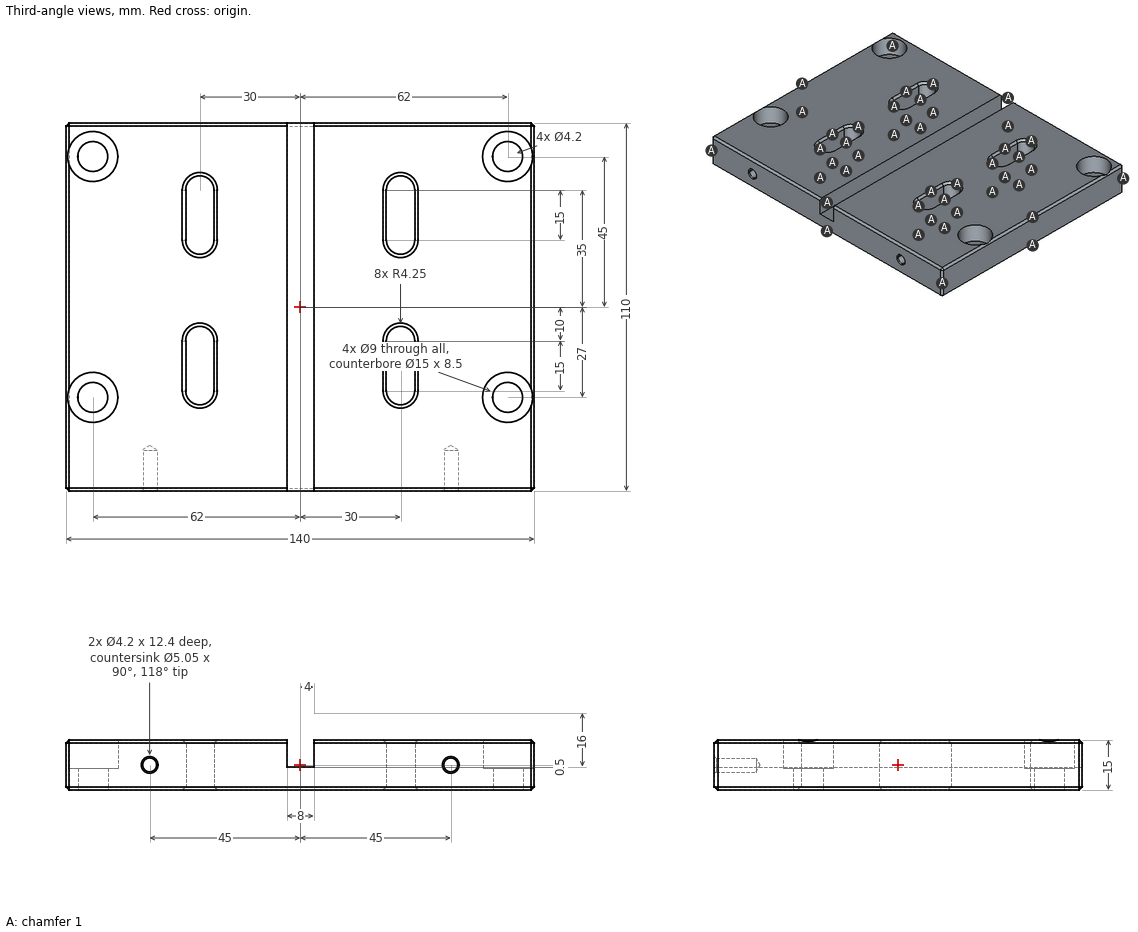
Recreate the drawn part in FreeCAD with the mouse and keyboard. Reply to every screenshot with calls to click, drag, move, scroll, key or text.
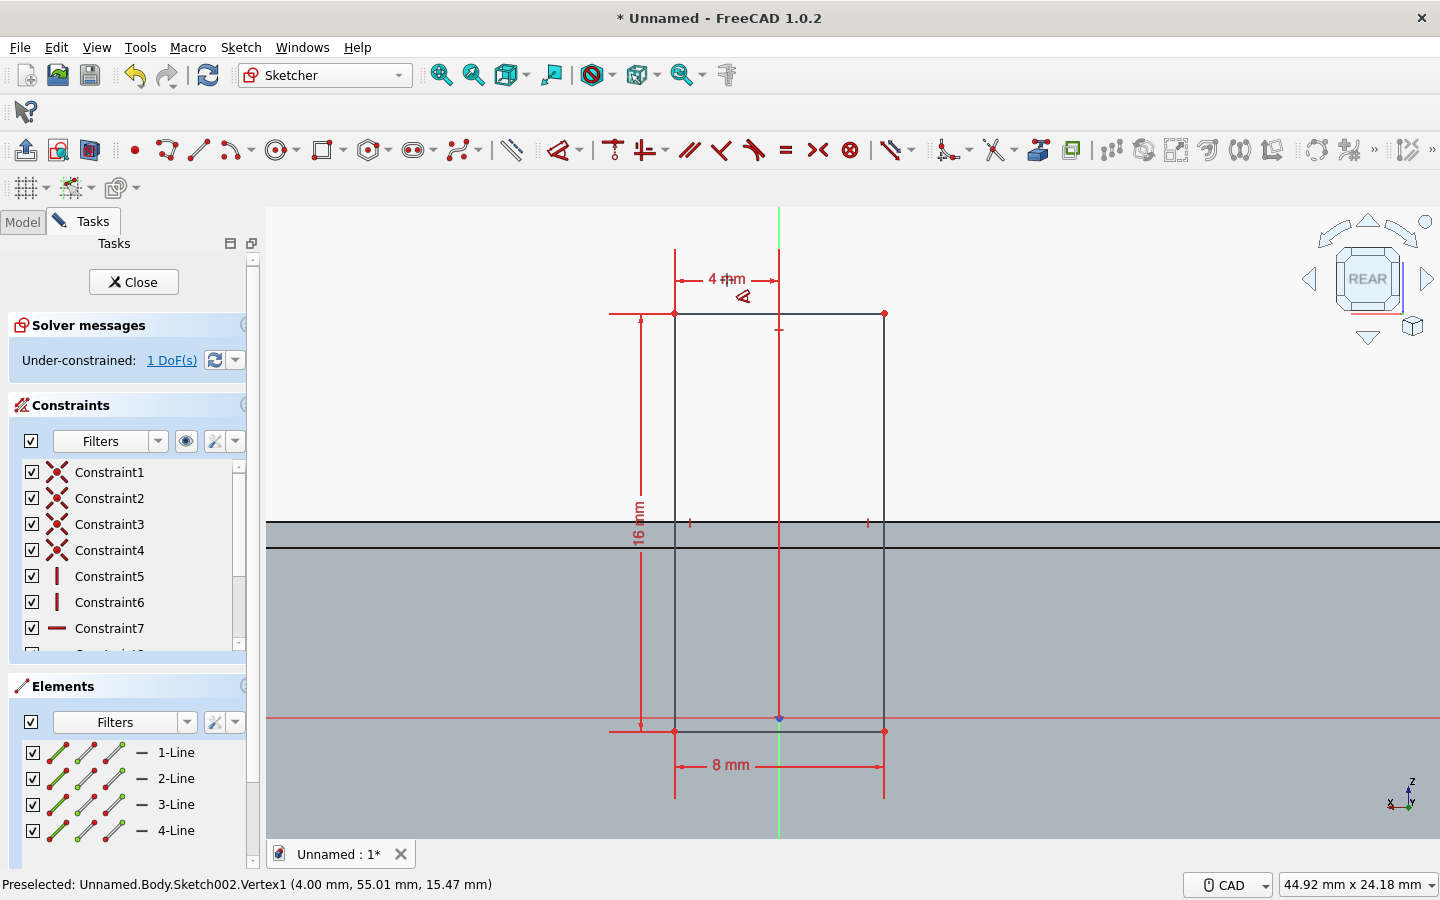
scroll(675, 732, up, 6)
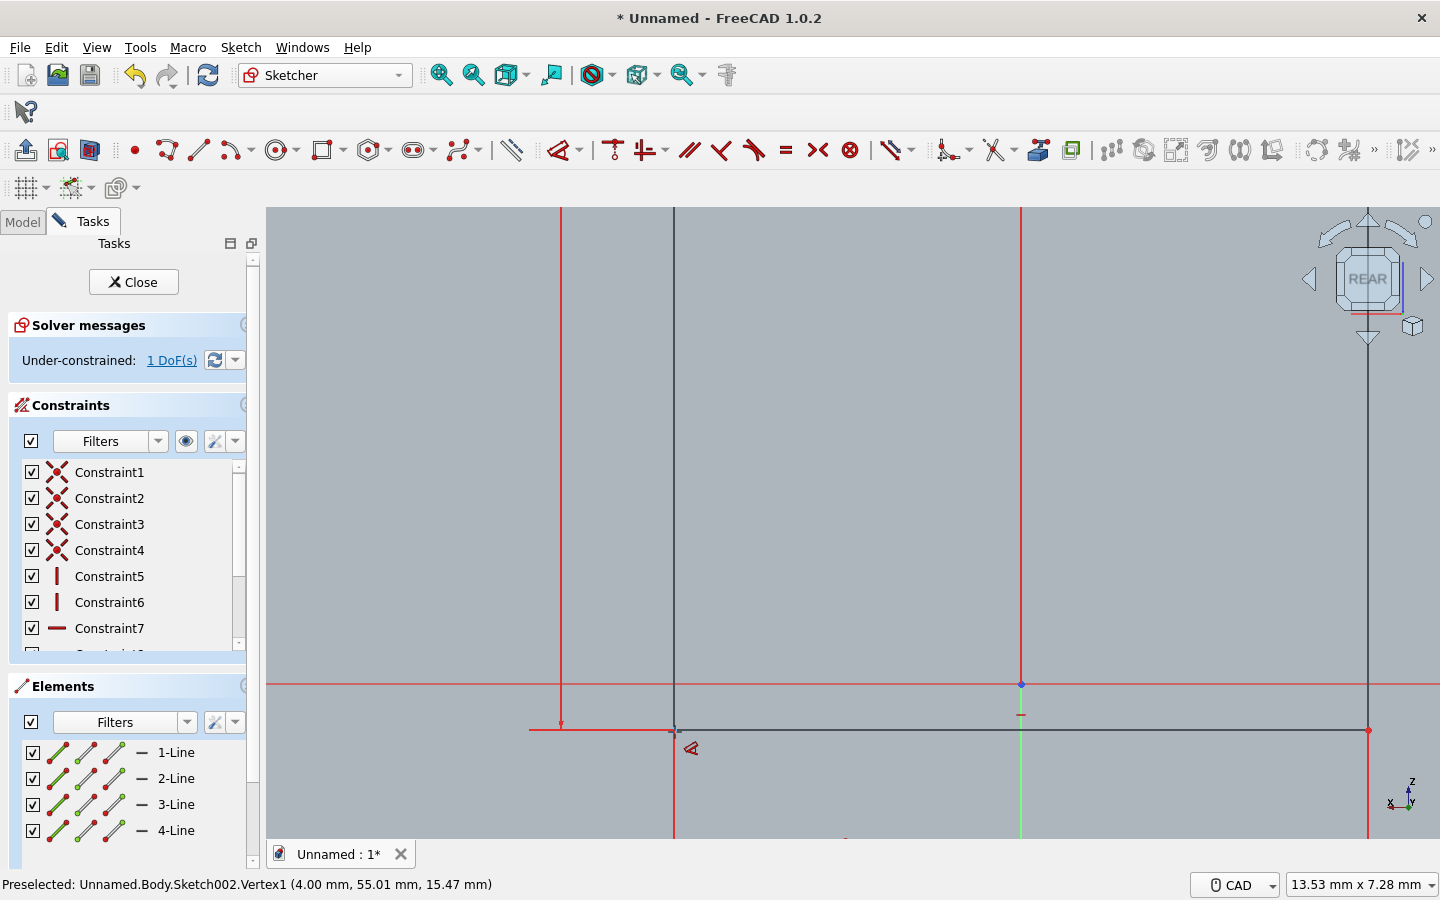
click(674, 730)
click(640, 707)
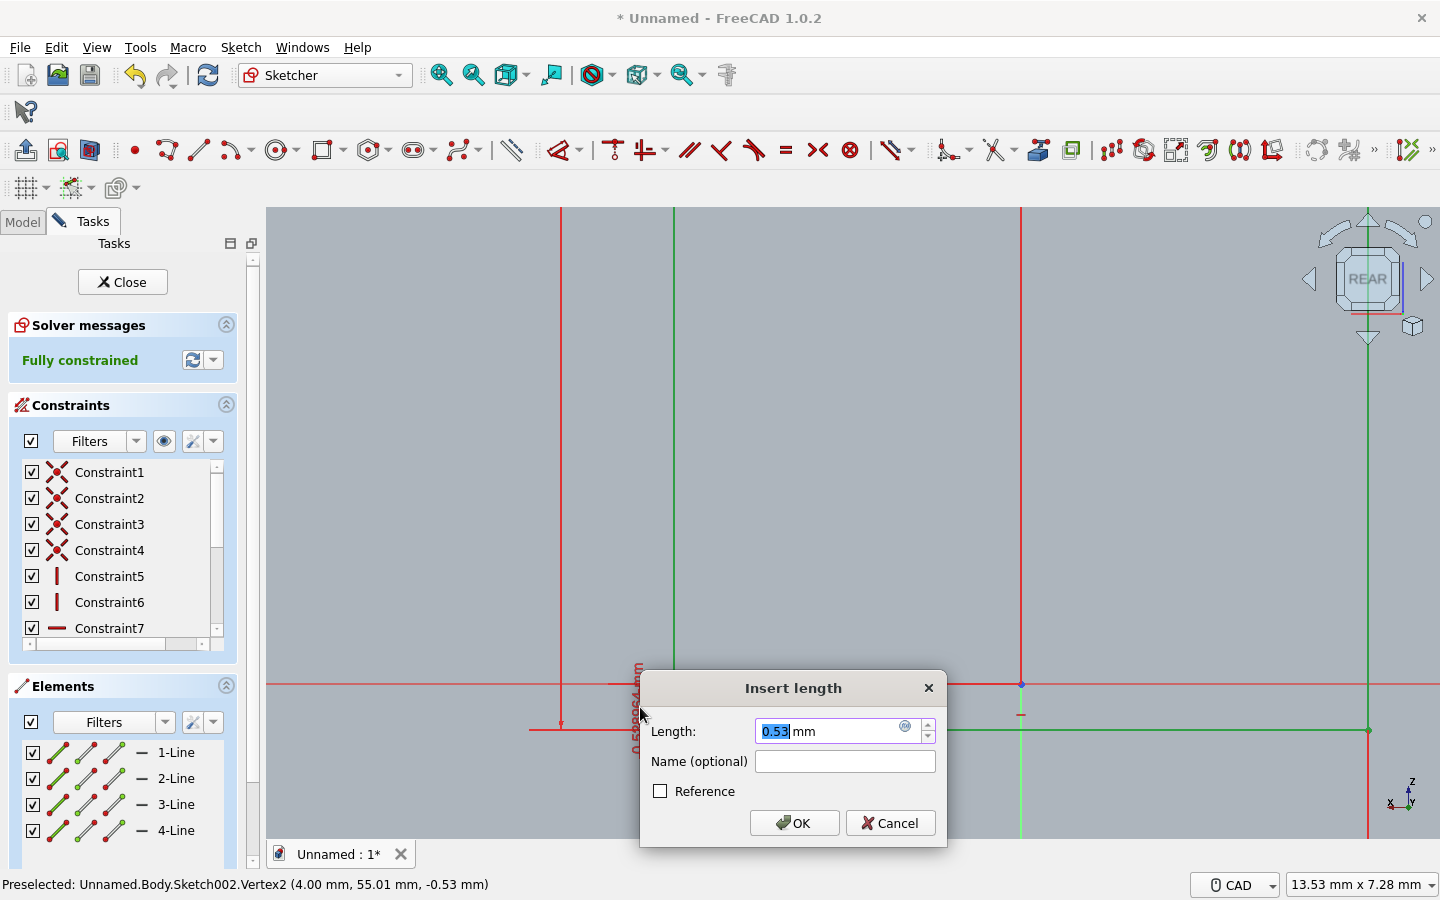
text(0.5)
key(Return)
key(Escape)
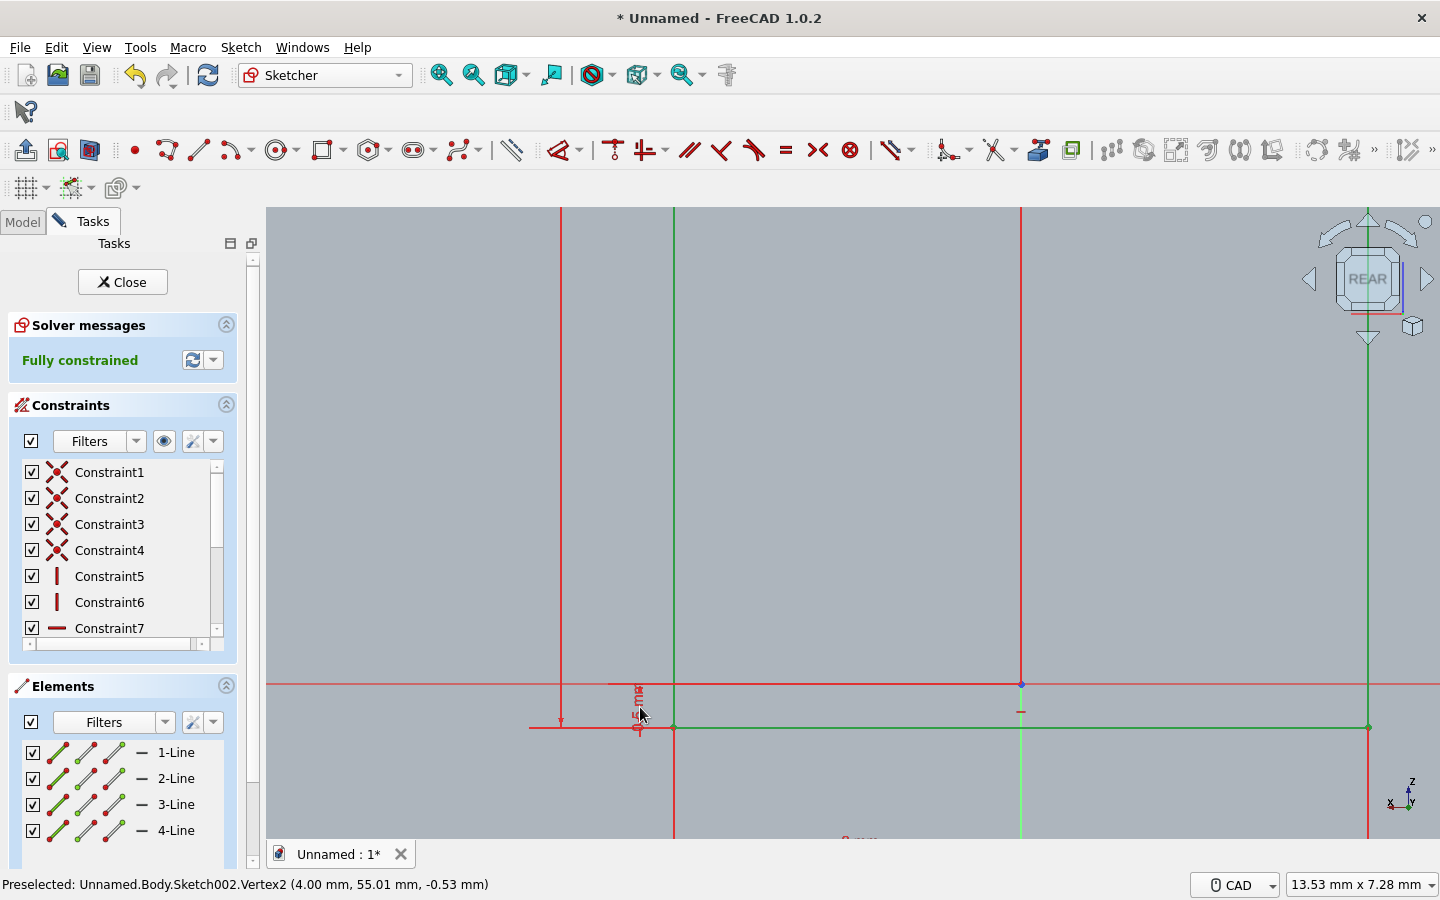
click(123, 282)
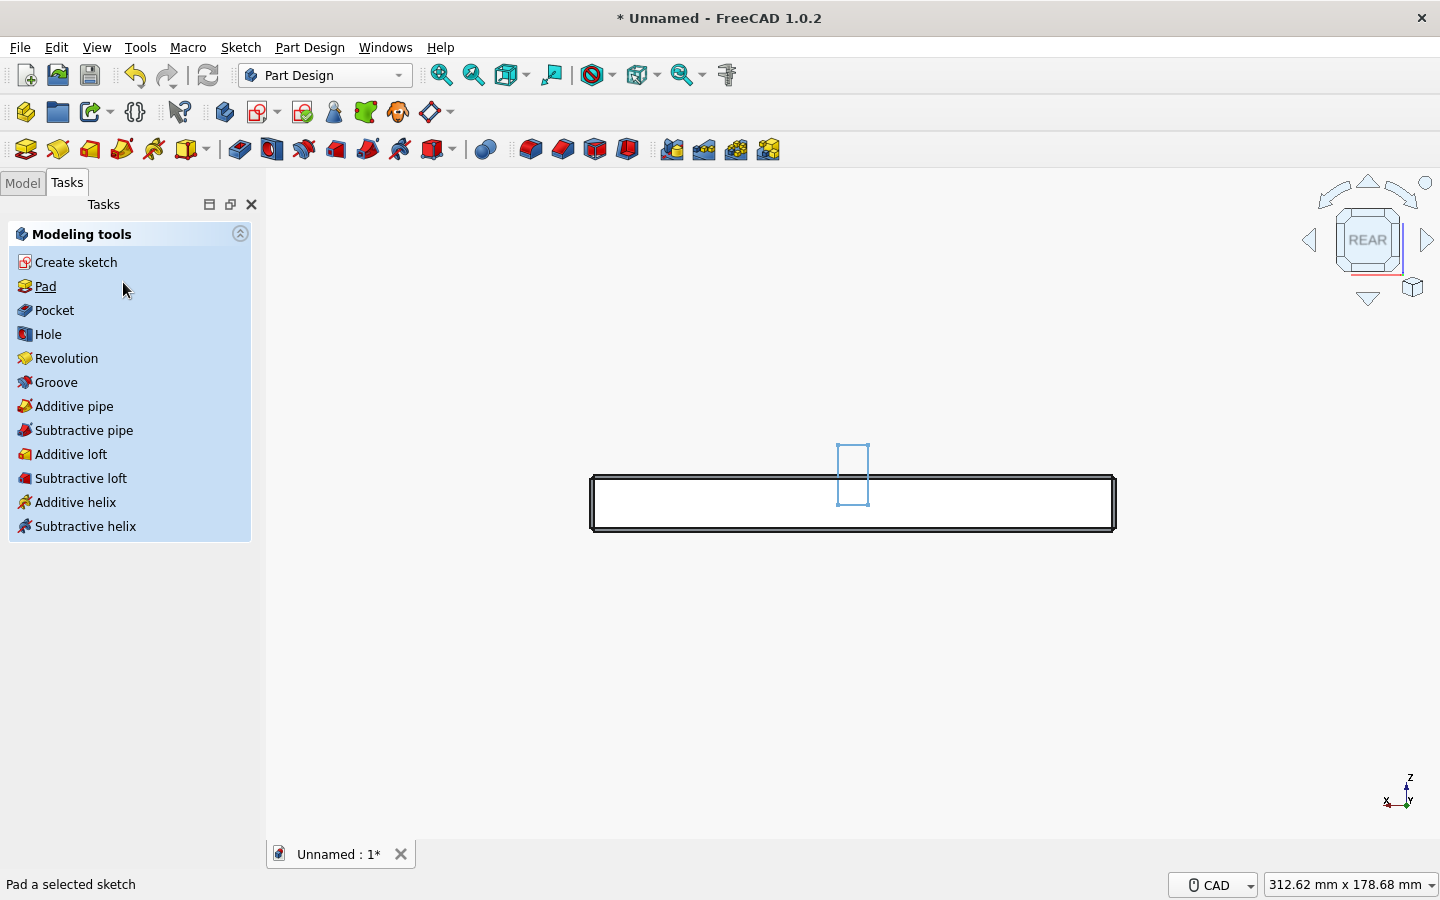
click(240, 150)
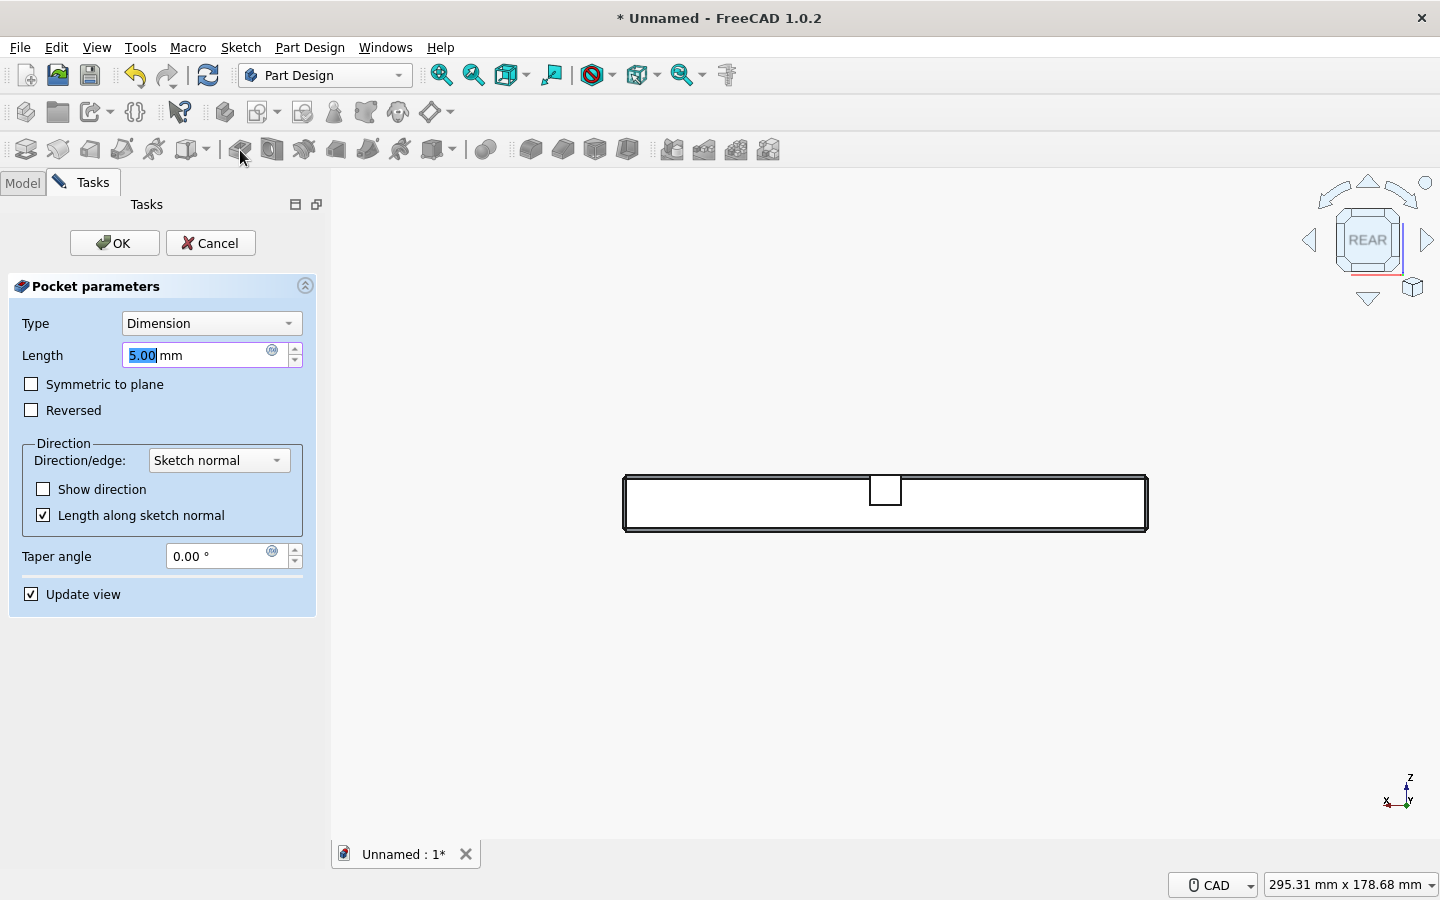
click(212, 324)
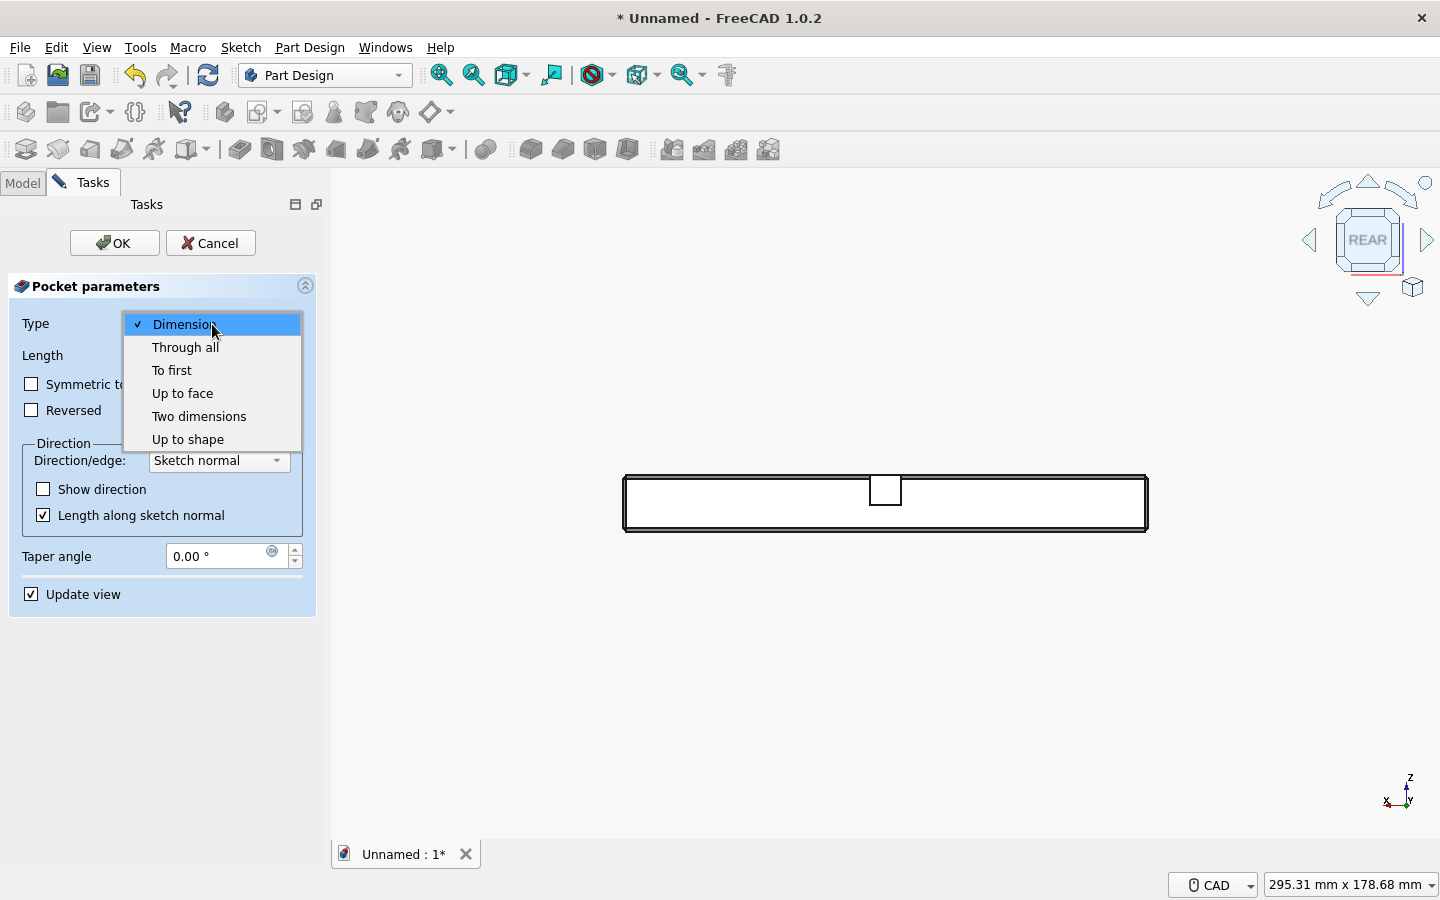
click(212, 348)